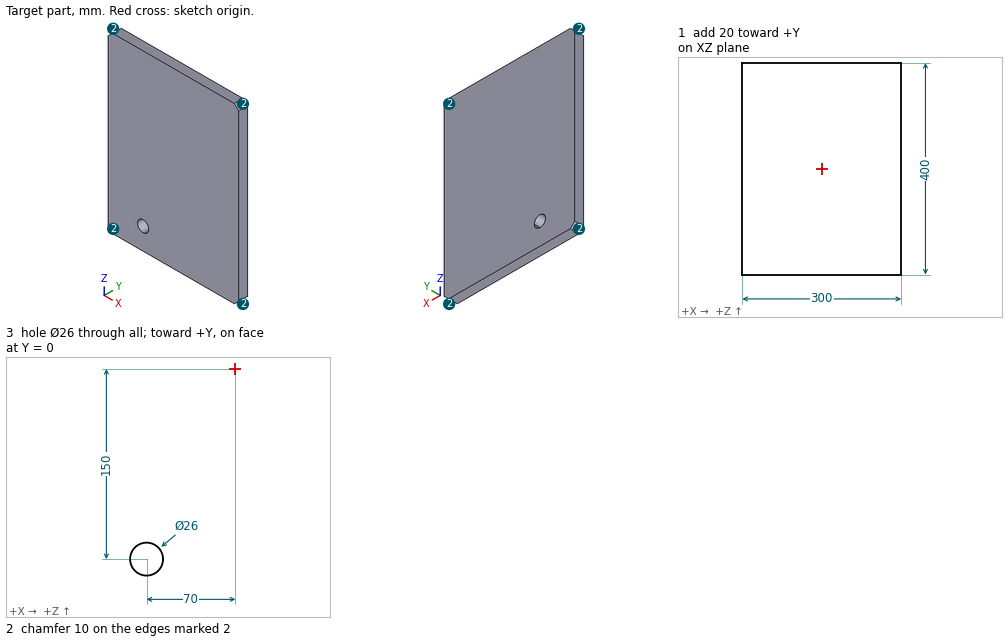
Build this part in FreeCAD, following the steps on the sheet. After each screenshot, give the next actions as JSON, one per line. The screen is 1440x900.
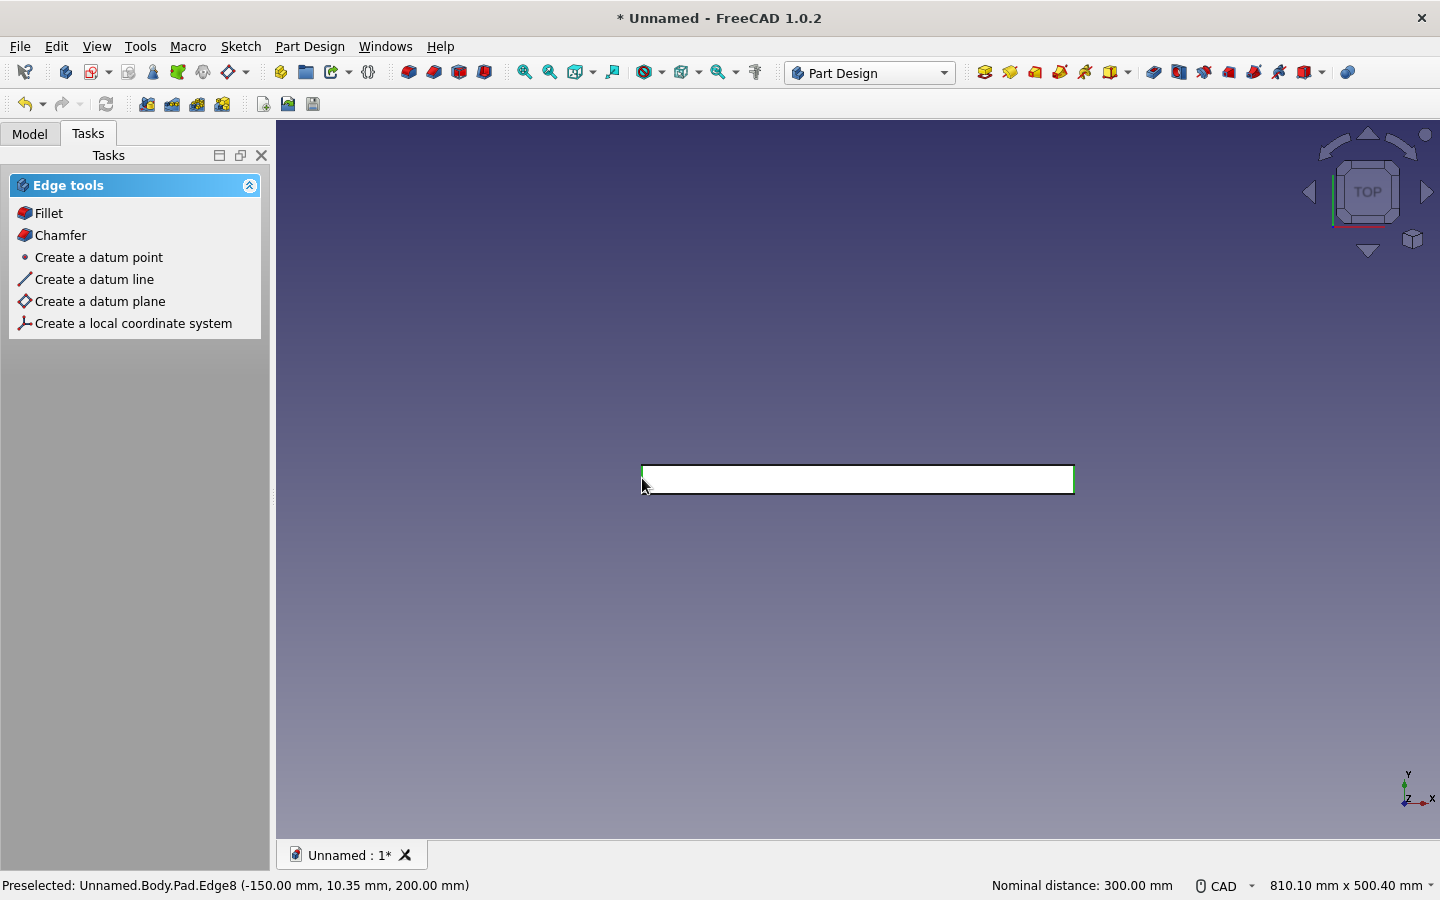
{"action": "key", "text": "1"}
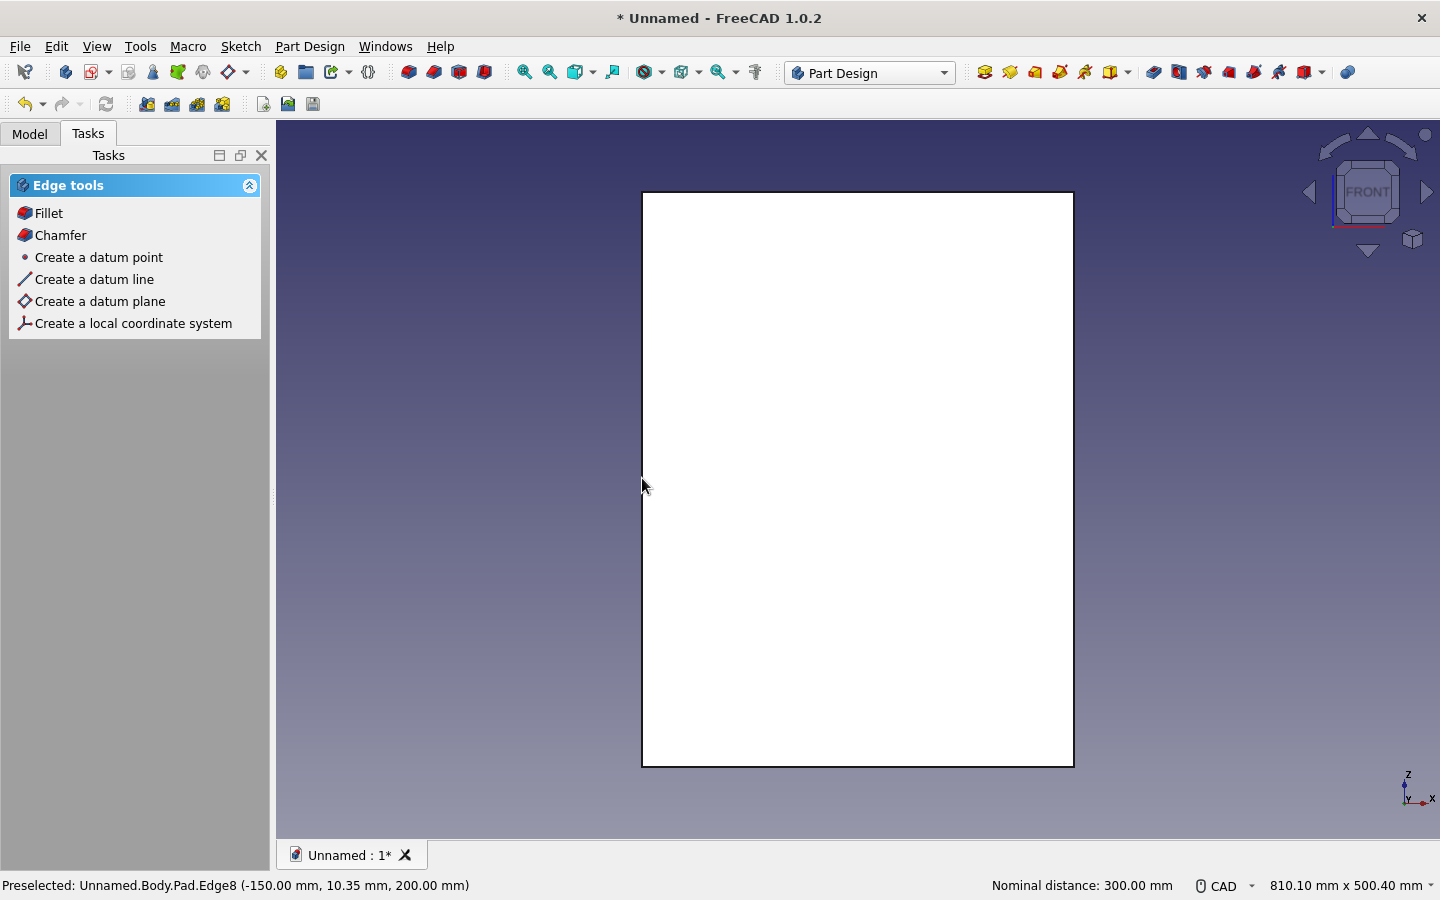
{"action": "key", "text": "3"}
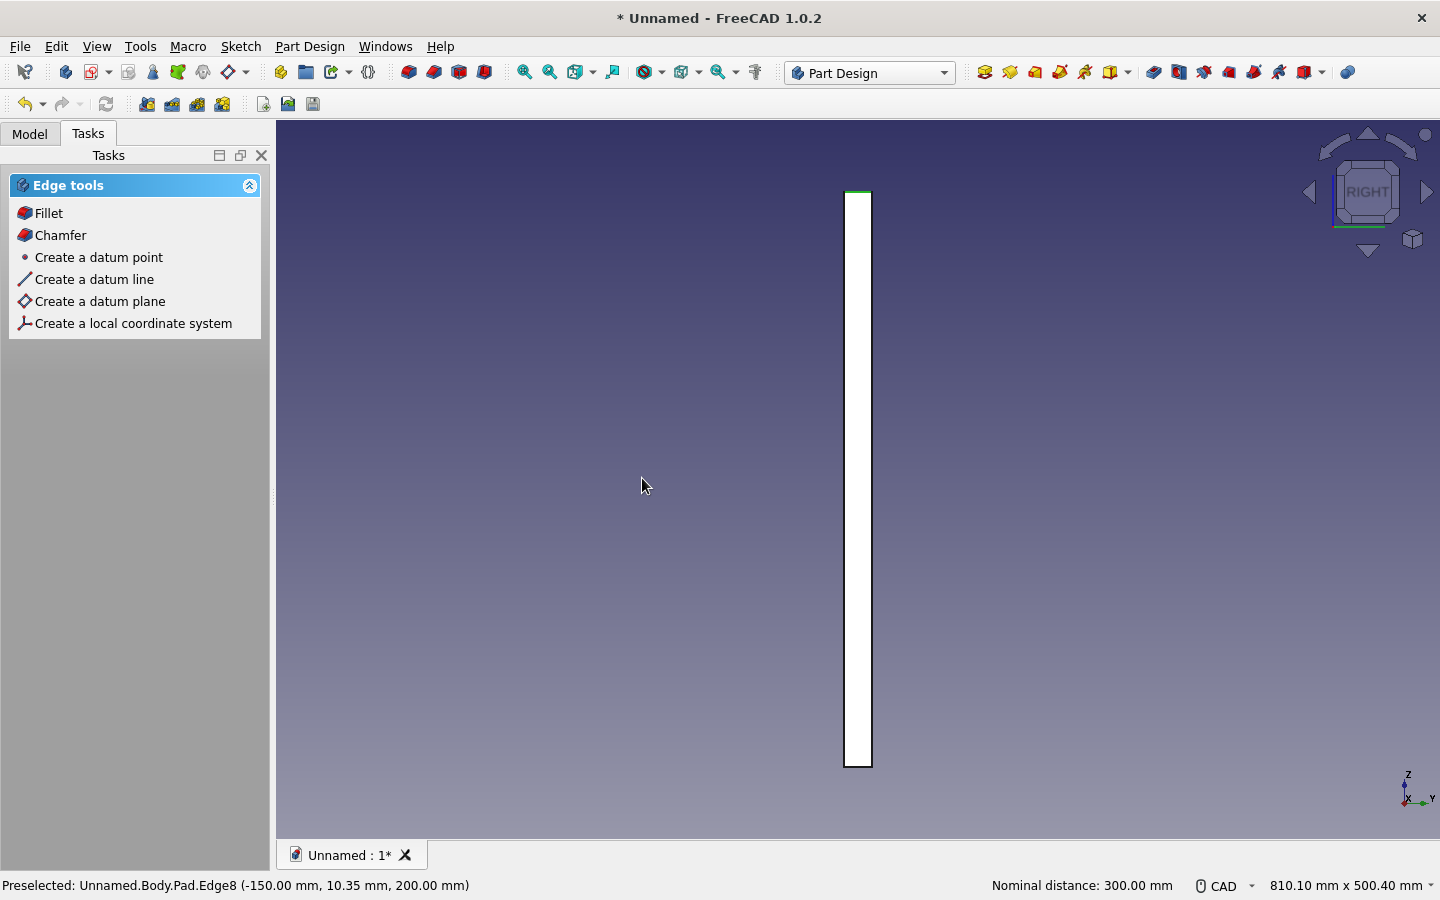
{"action": "left_click", "coordinate": [858, 766], "text": "ctrl"}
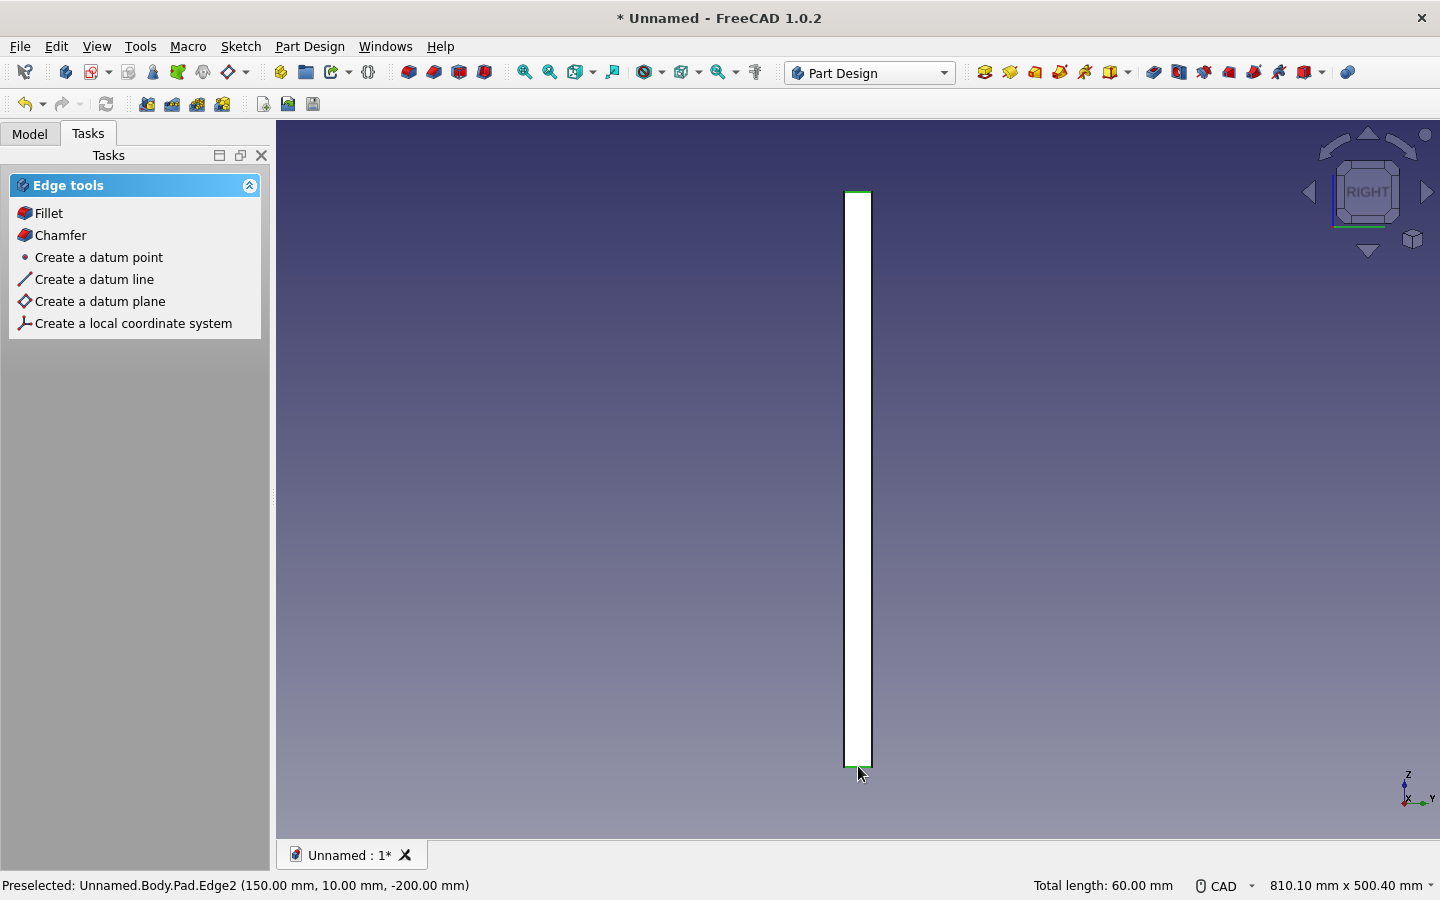
{"action": "key", "text": "5"}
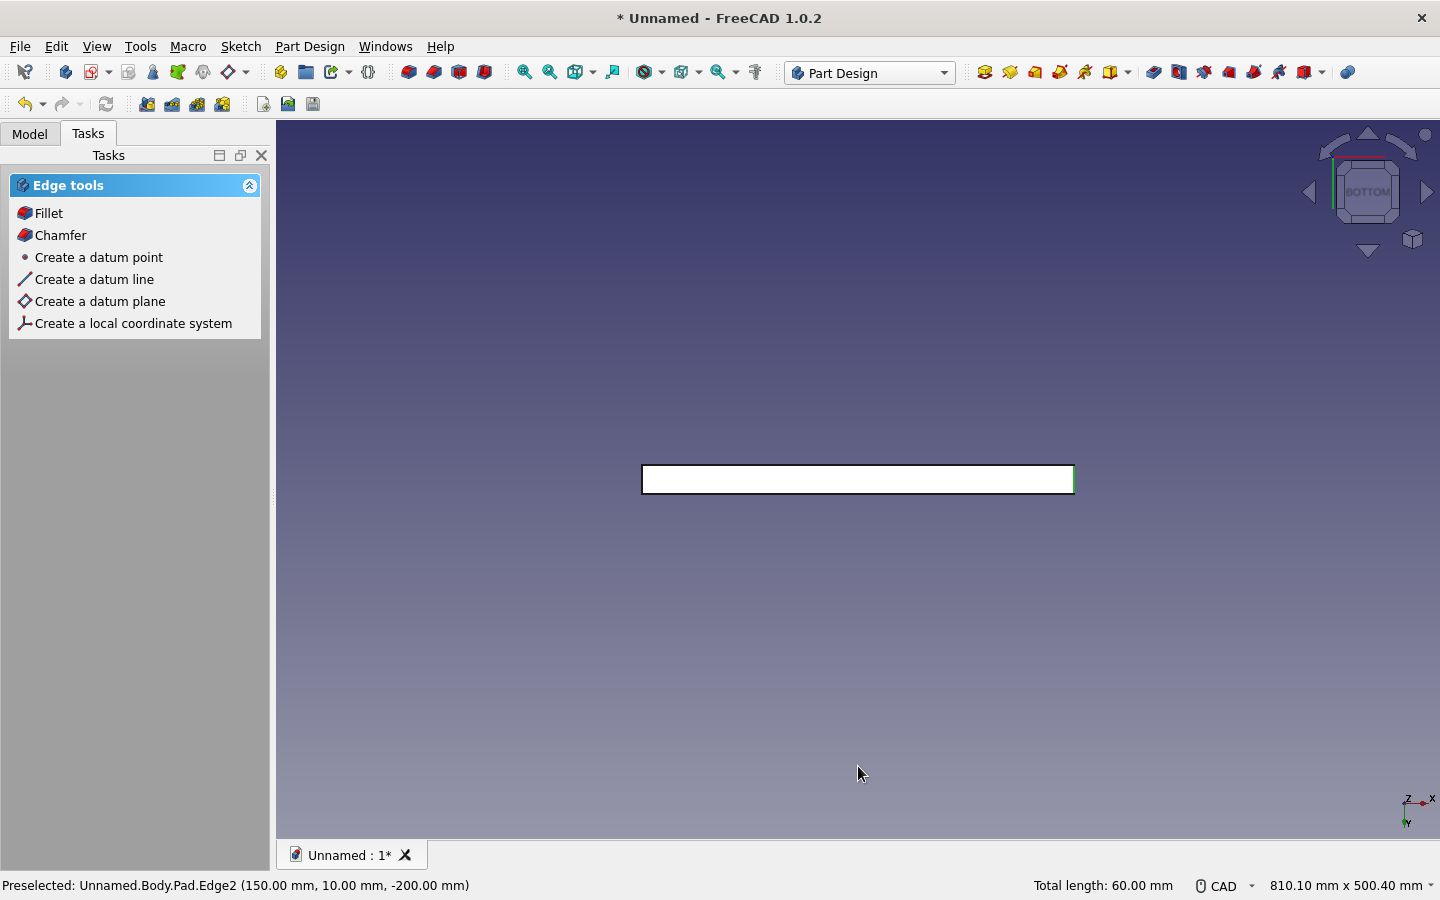
{"action": "left_click", "coordinate": [525, 72]}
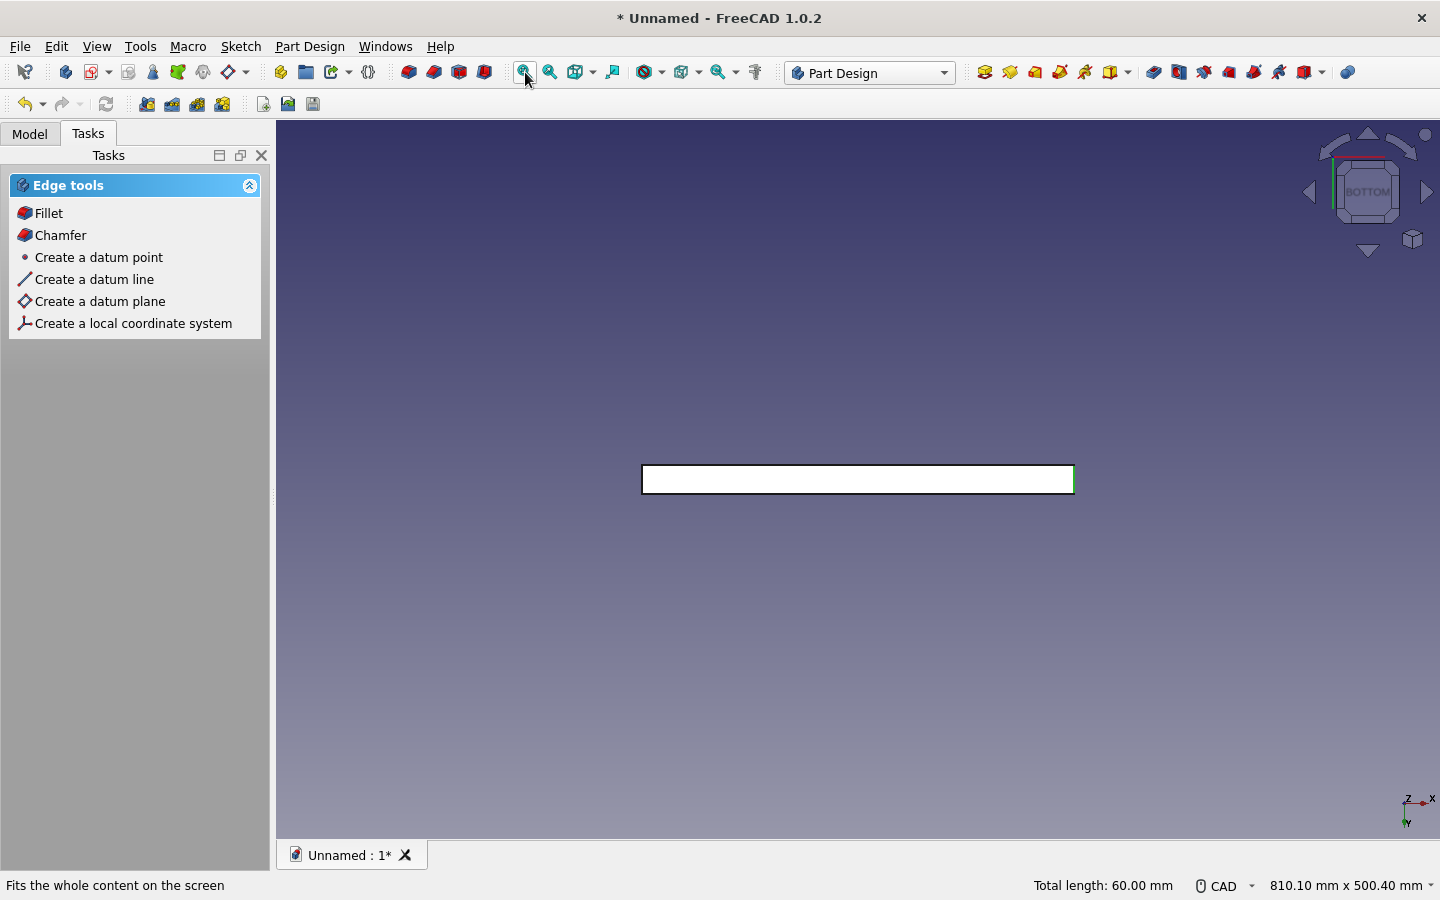
{"action": "left_click", "coordinate": [642, 478], "text": "ctrl"}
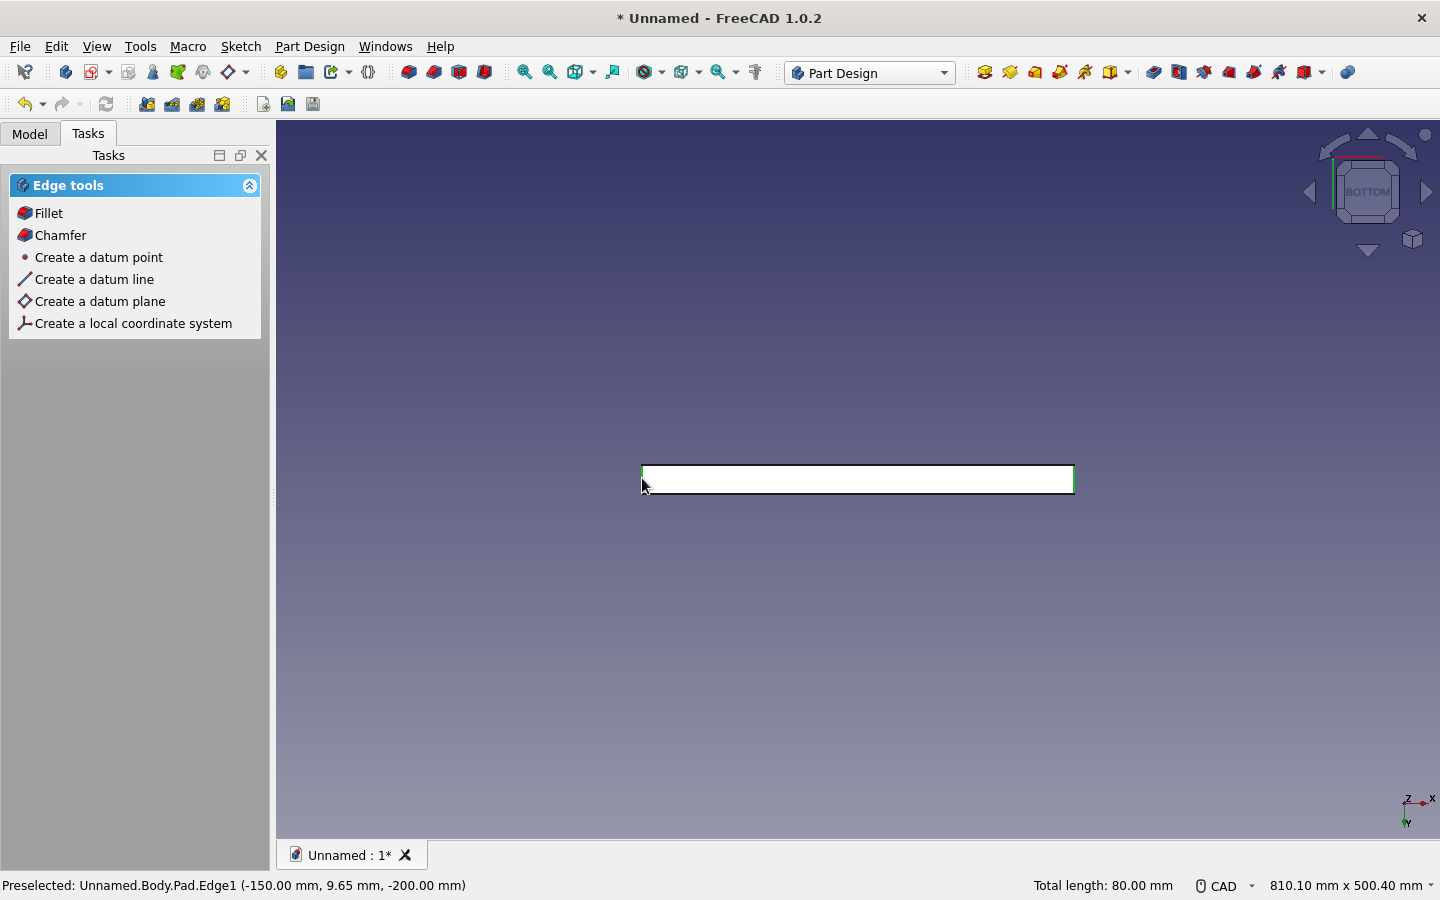
{"action": "left_click", "coordinate": [434, 72]}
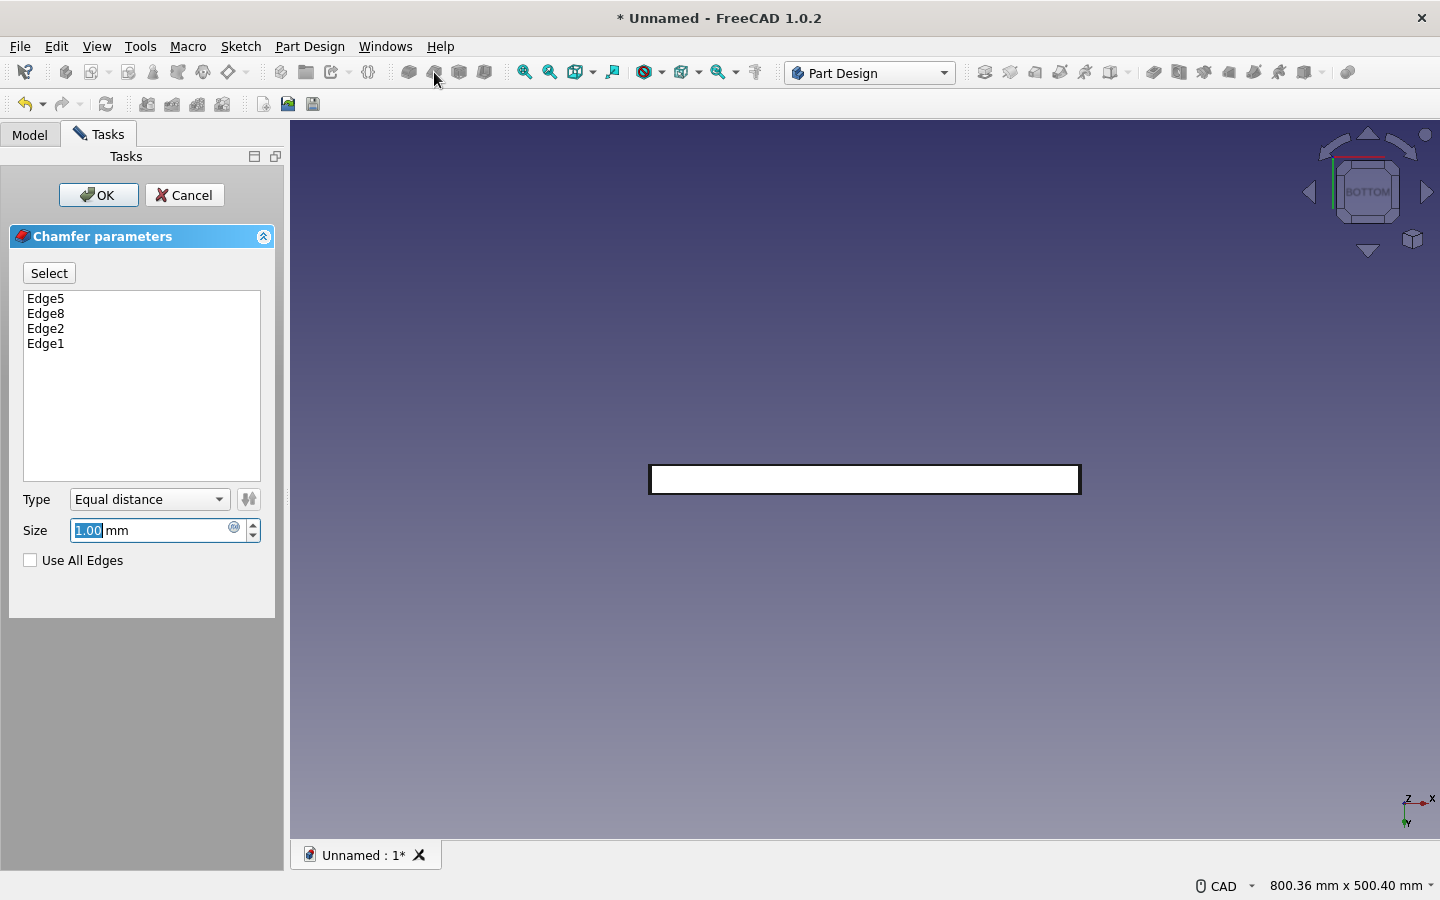
{"action": "type", "text": "10"}
{"action": "key", "text": "Tab"}